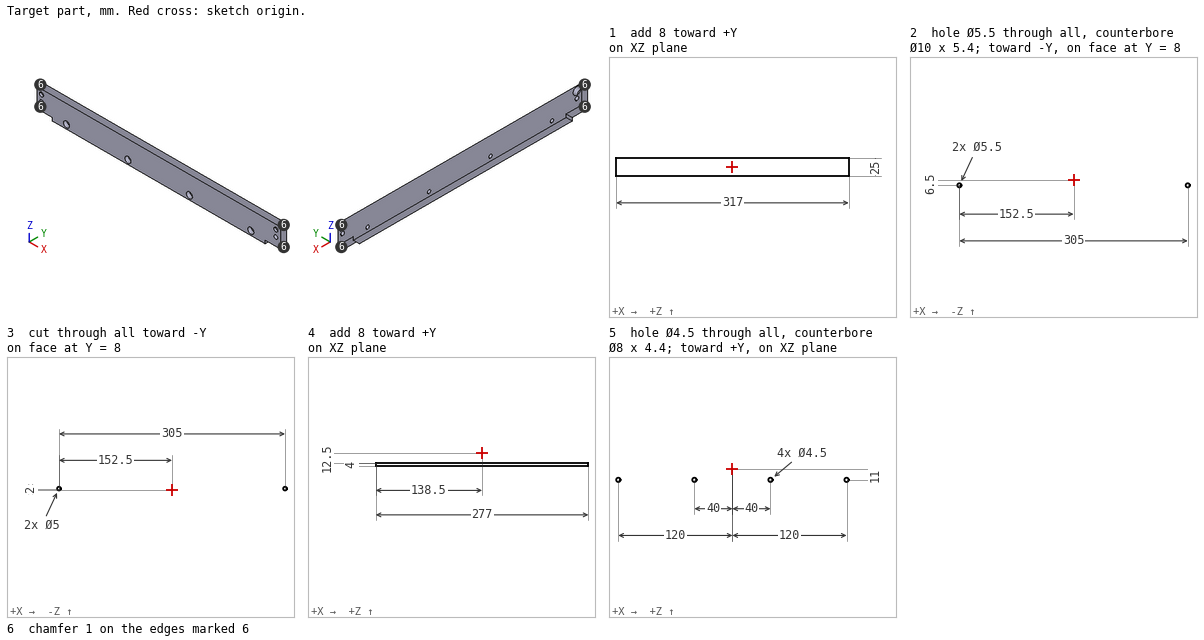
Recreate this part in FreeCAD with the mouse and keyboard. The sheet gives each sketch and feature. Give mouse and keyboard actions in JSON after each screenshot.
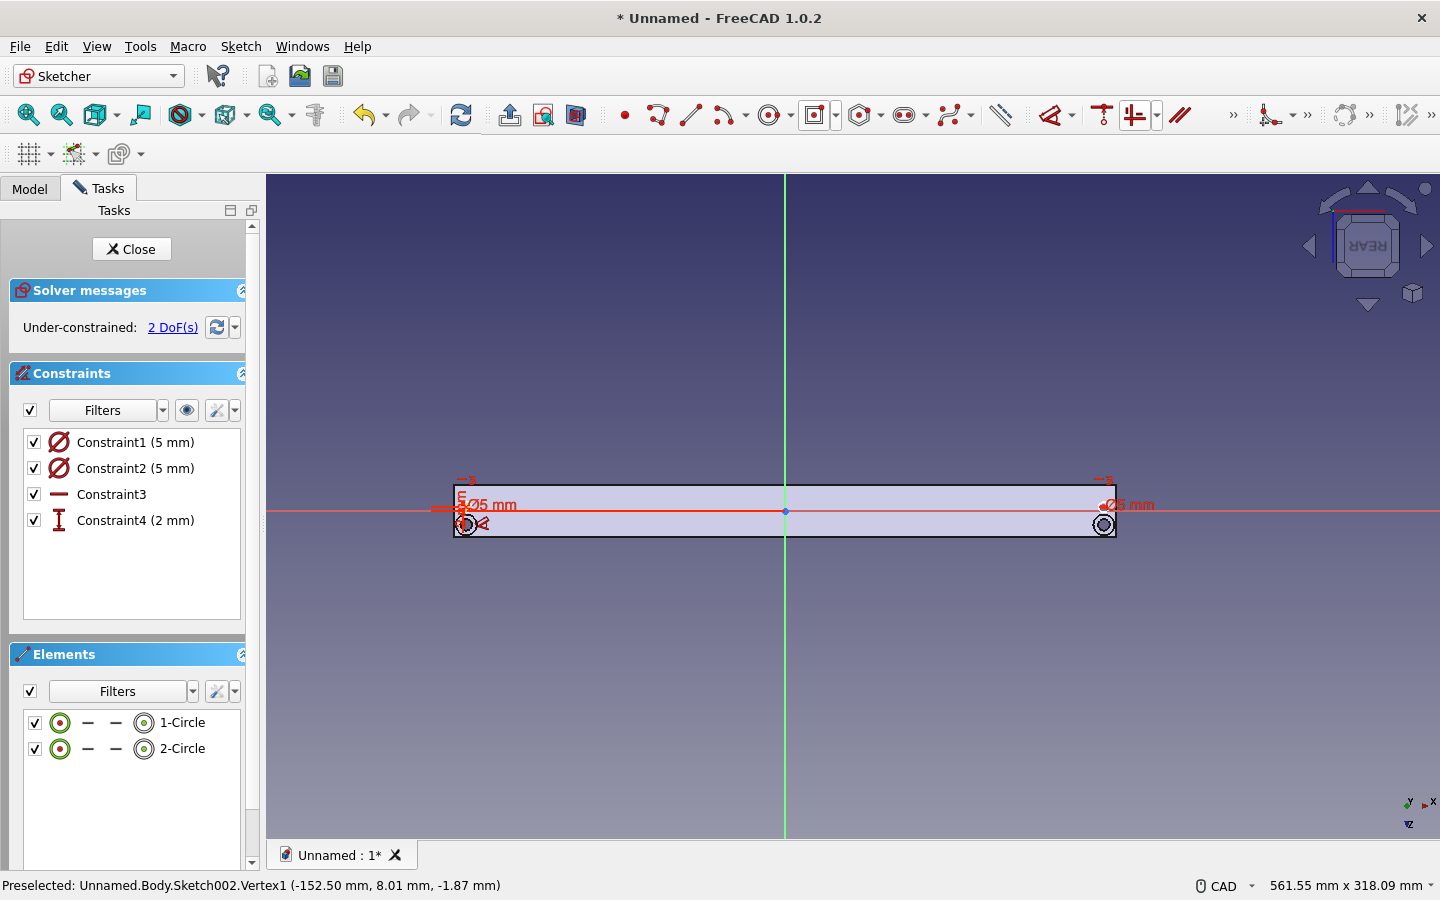
{"action": "left_click", "coordinate": [466, 507]}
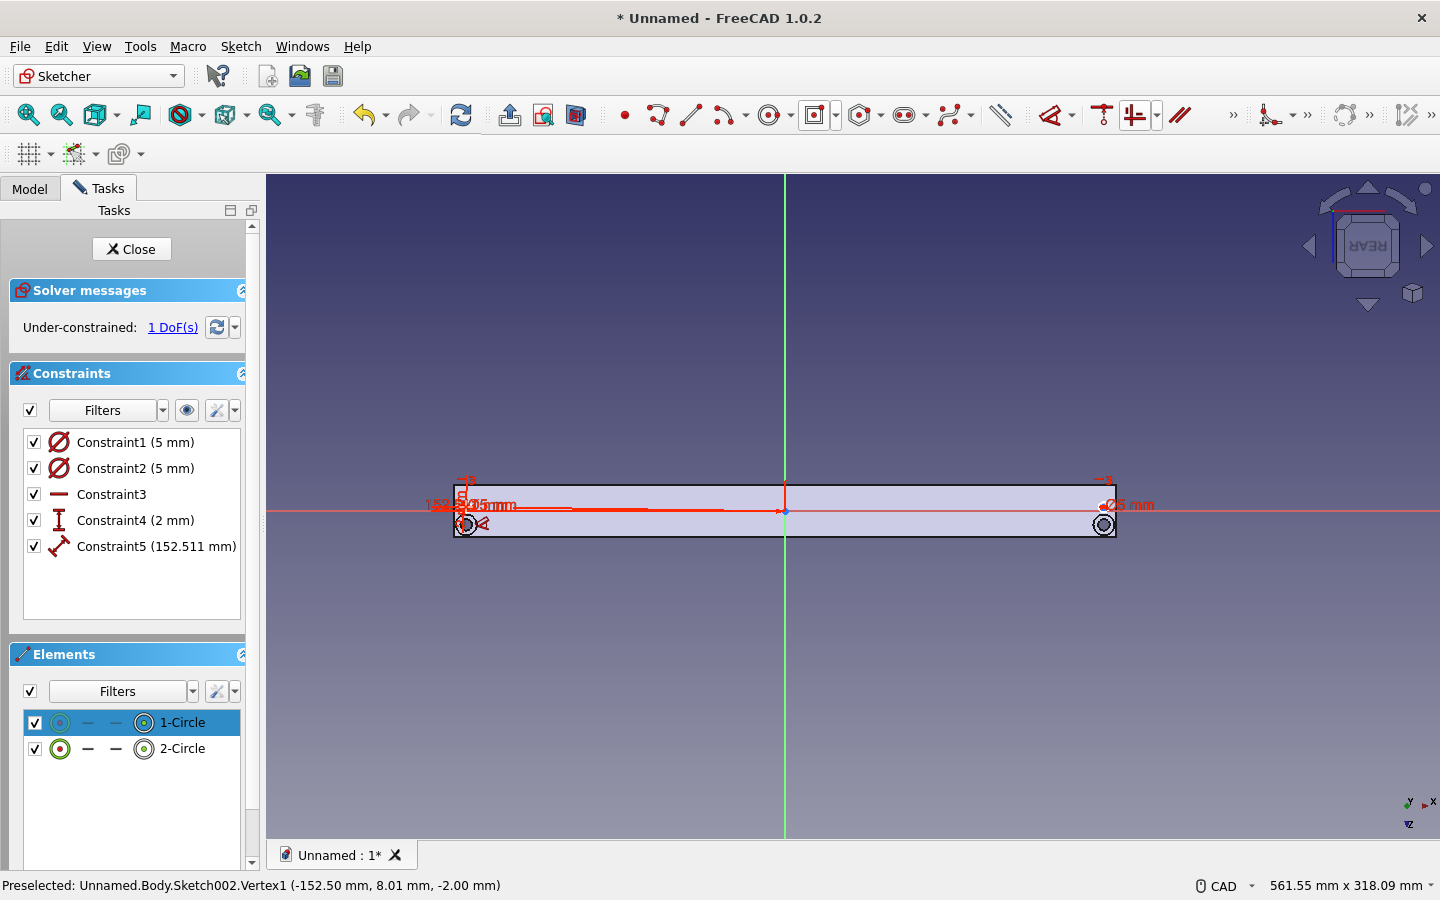
{"action": "left_click", "coordinate": [1104, 507]}
{"action": "left_click", "coordinate": [638, 541]}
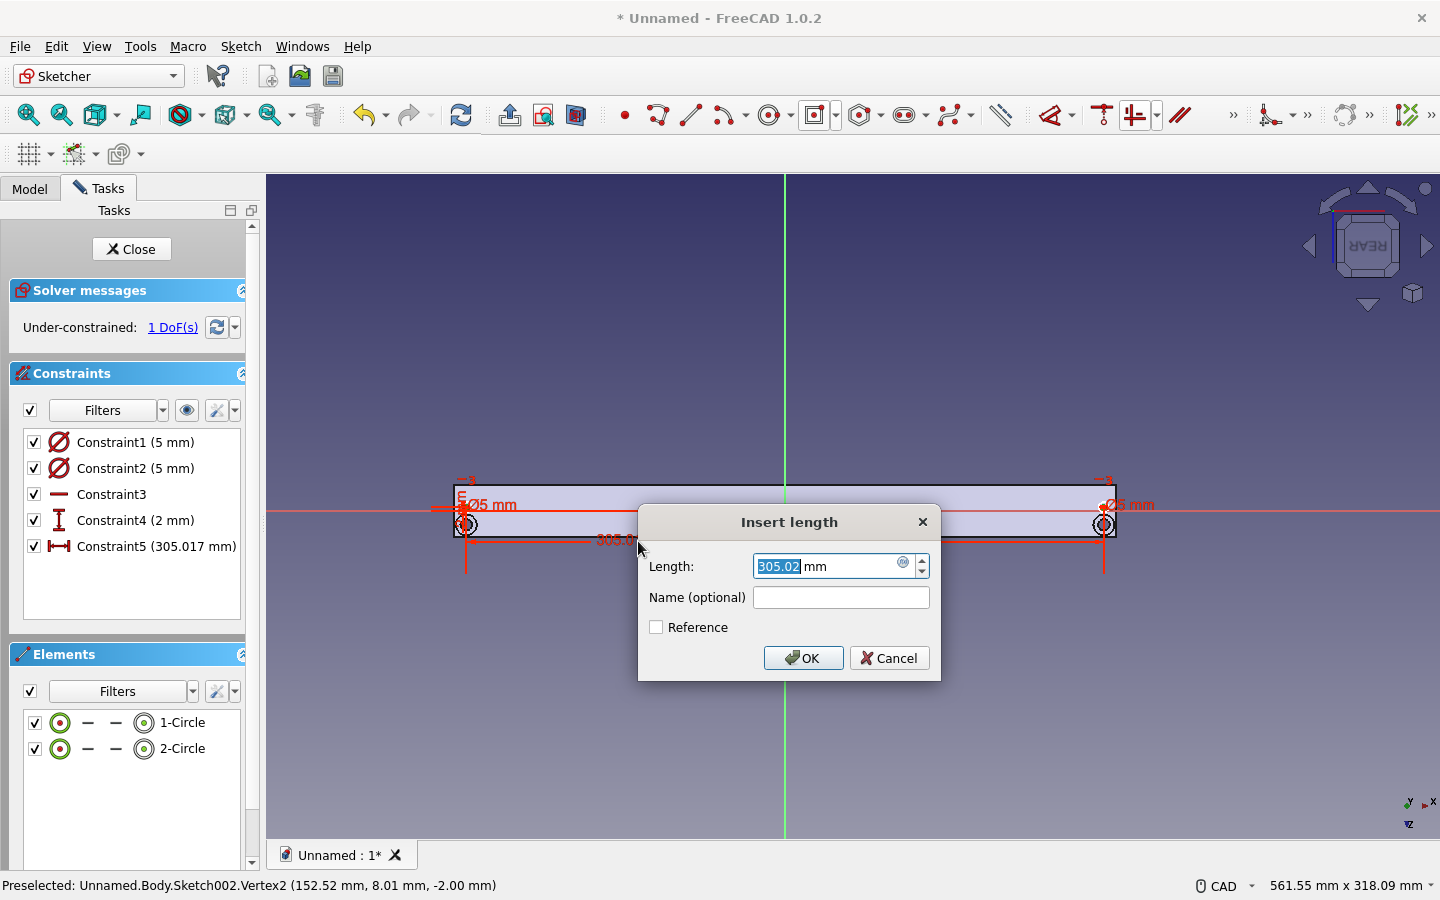
{"action": "type", "text": "305"}
{"action": "key", "text": "Return"}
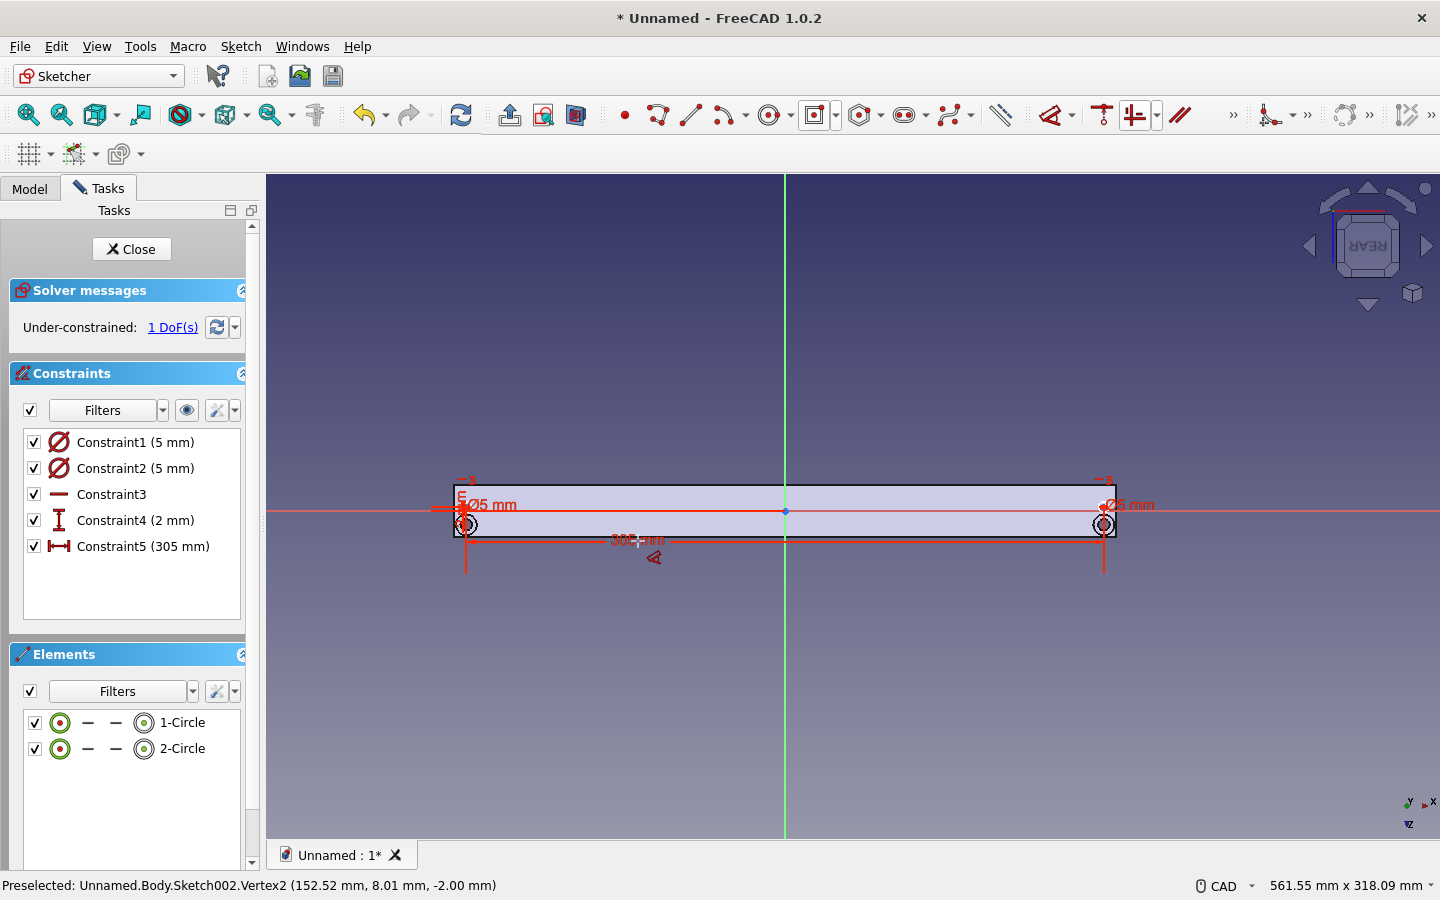
{"action": "left_click", "coordinate": [466, 507]}
{"action": "left_click", "coordinate": [552, 545]}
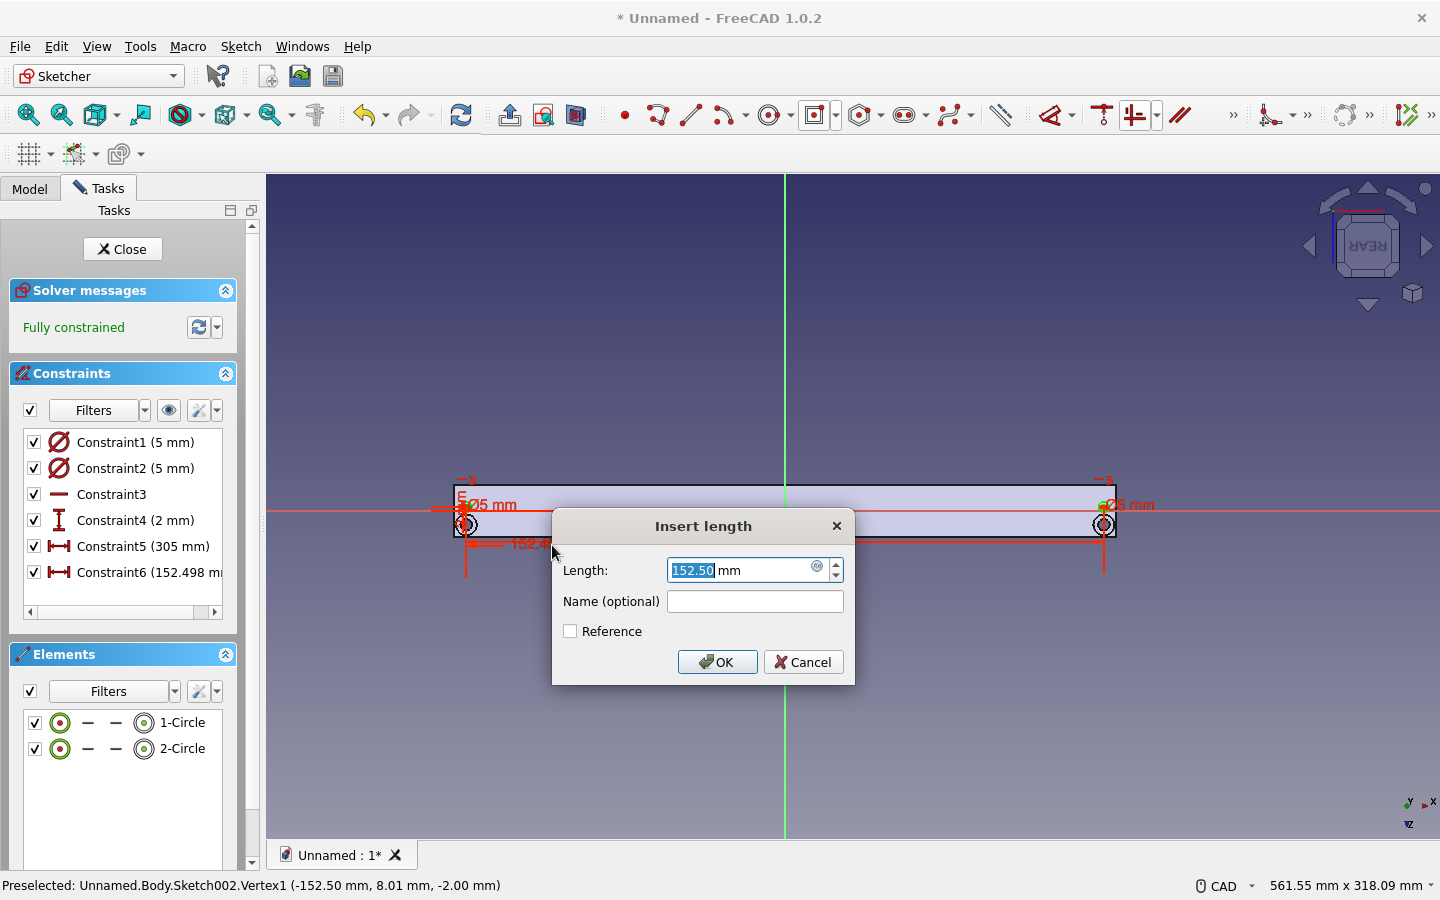
{"action": "type", "text": "152.5"}
{"action": "key", "text": "Return"}
{"action": "key", "text": "Escape"}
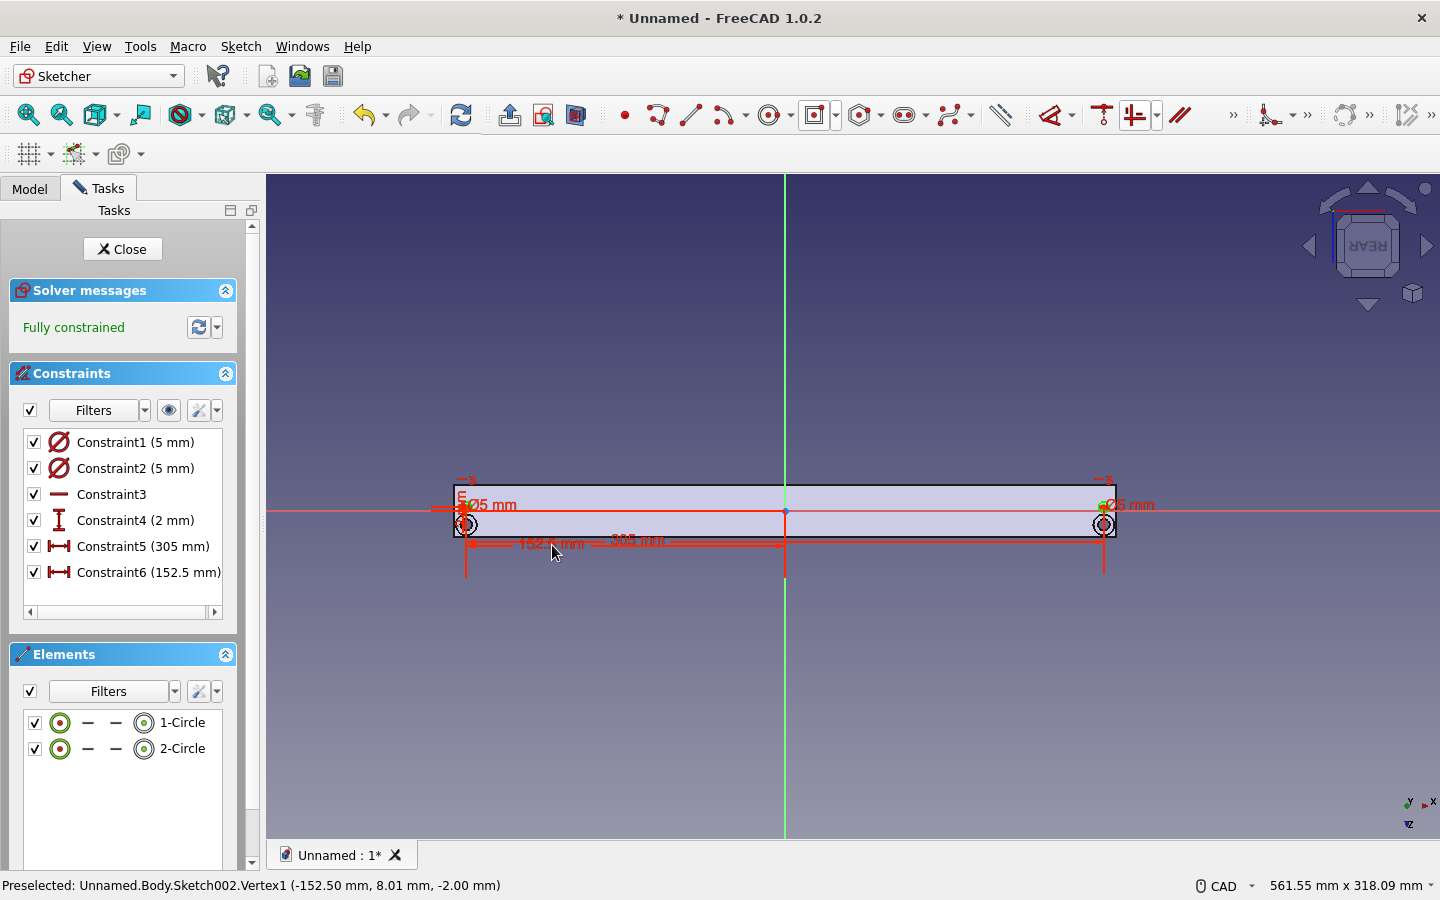
{"action": "left_click", "coordinate": [123, 249]}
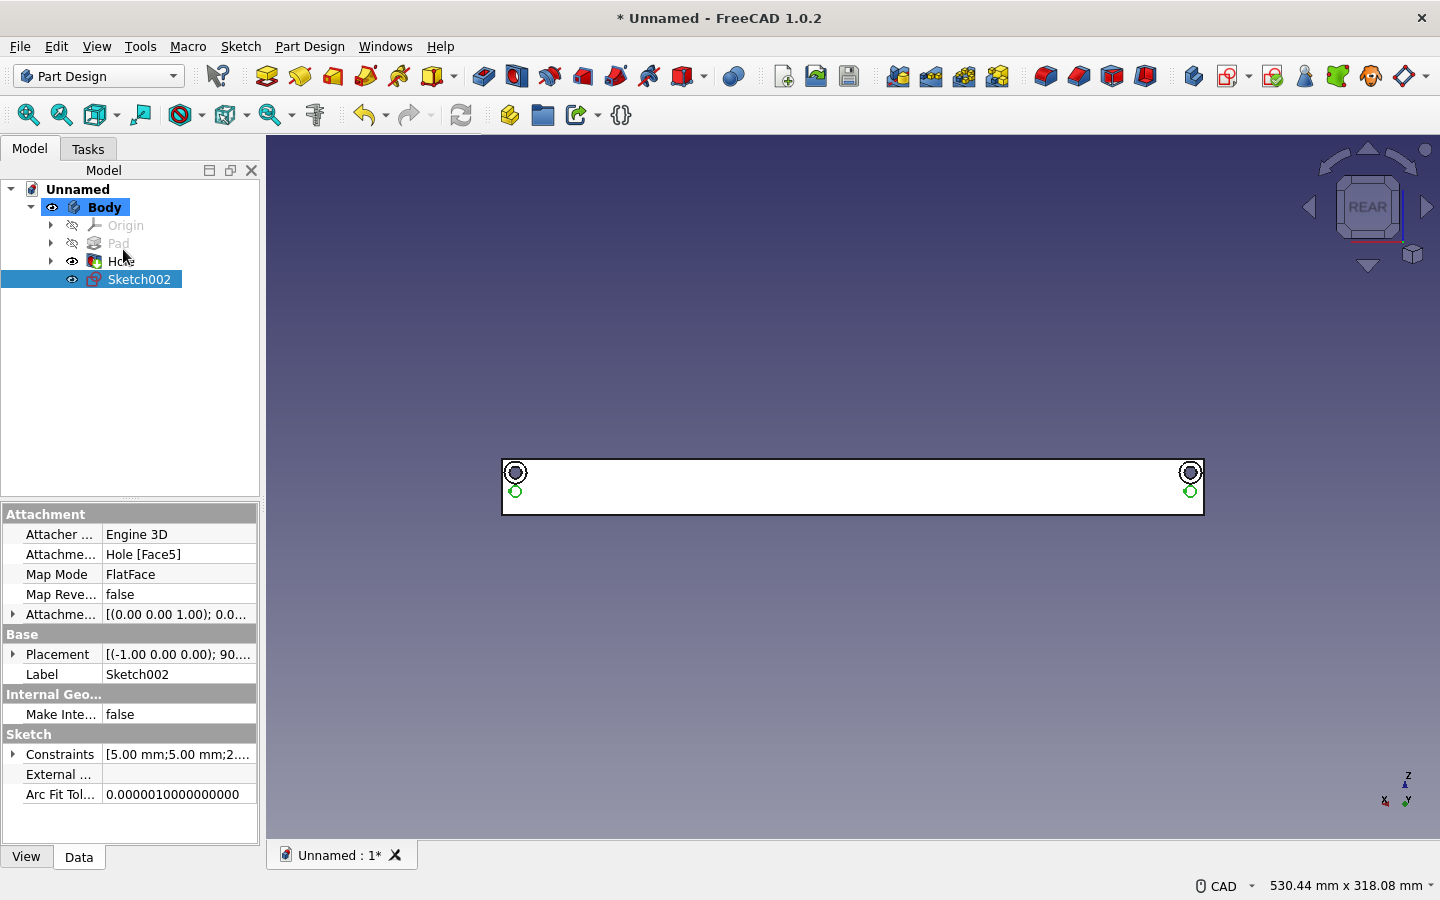
{"action": "left_click", "coordinate": [484, 76]}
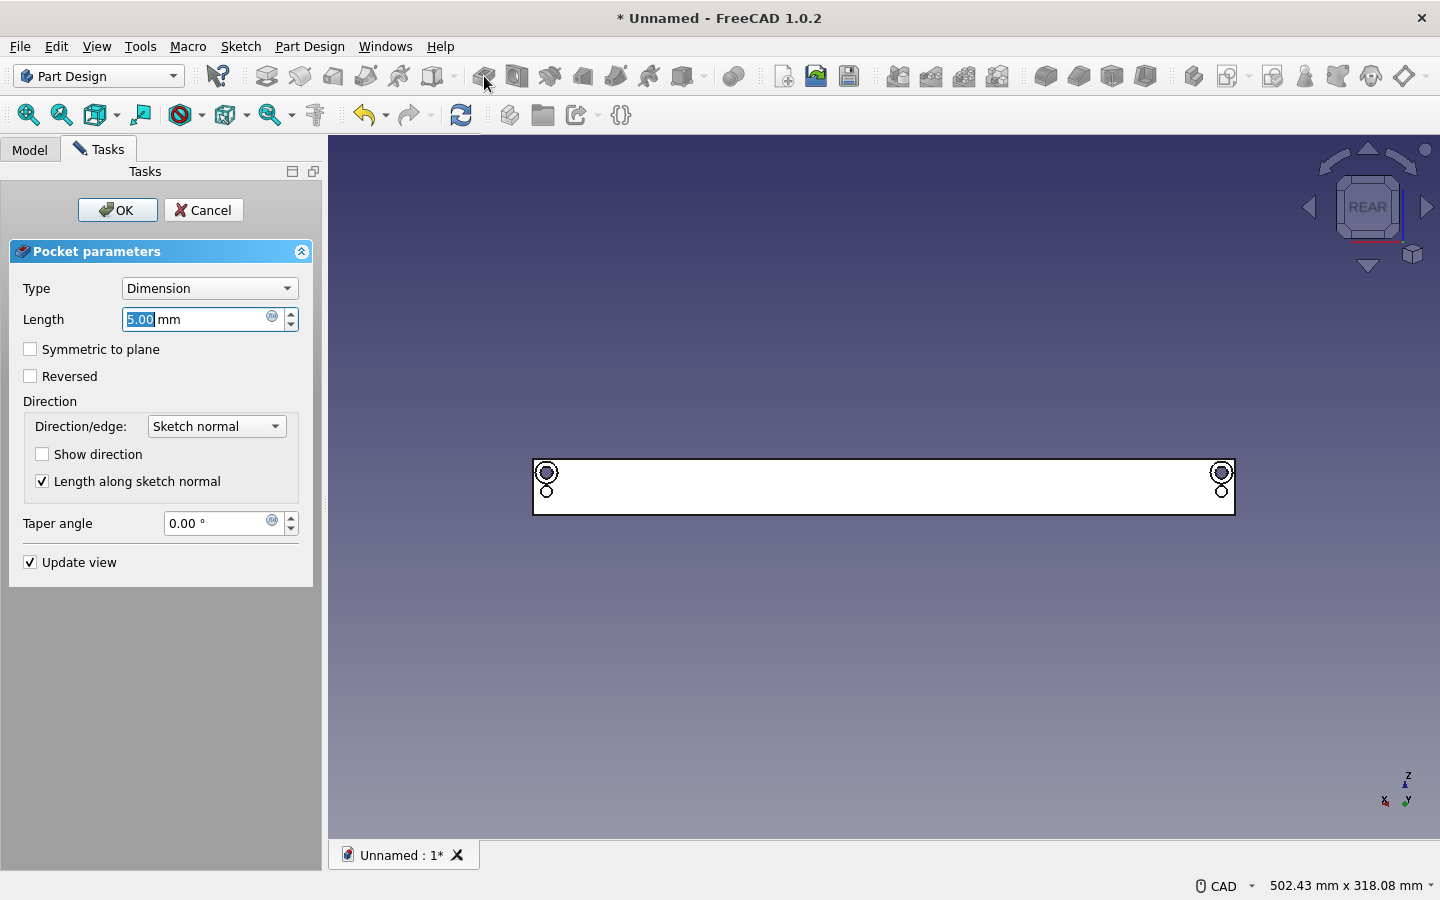
{"action": "left_click", "coordinate": [210, 288]}